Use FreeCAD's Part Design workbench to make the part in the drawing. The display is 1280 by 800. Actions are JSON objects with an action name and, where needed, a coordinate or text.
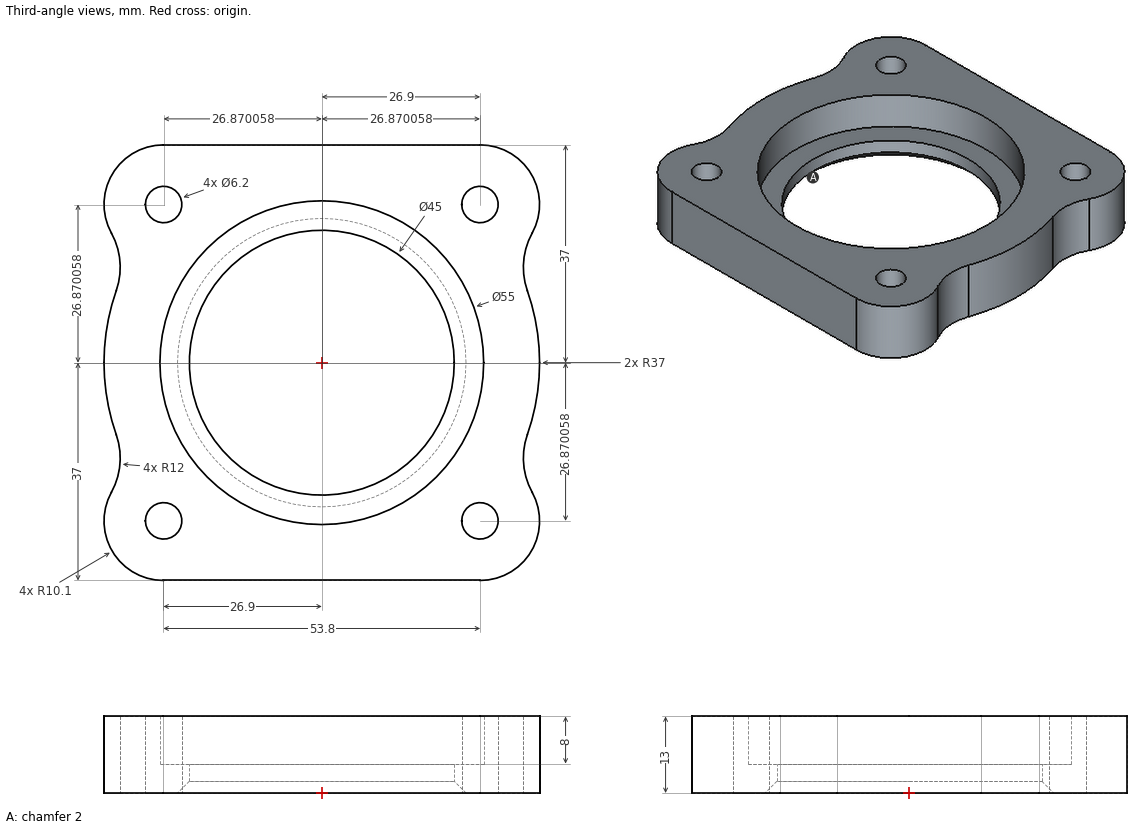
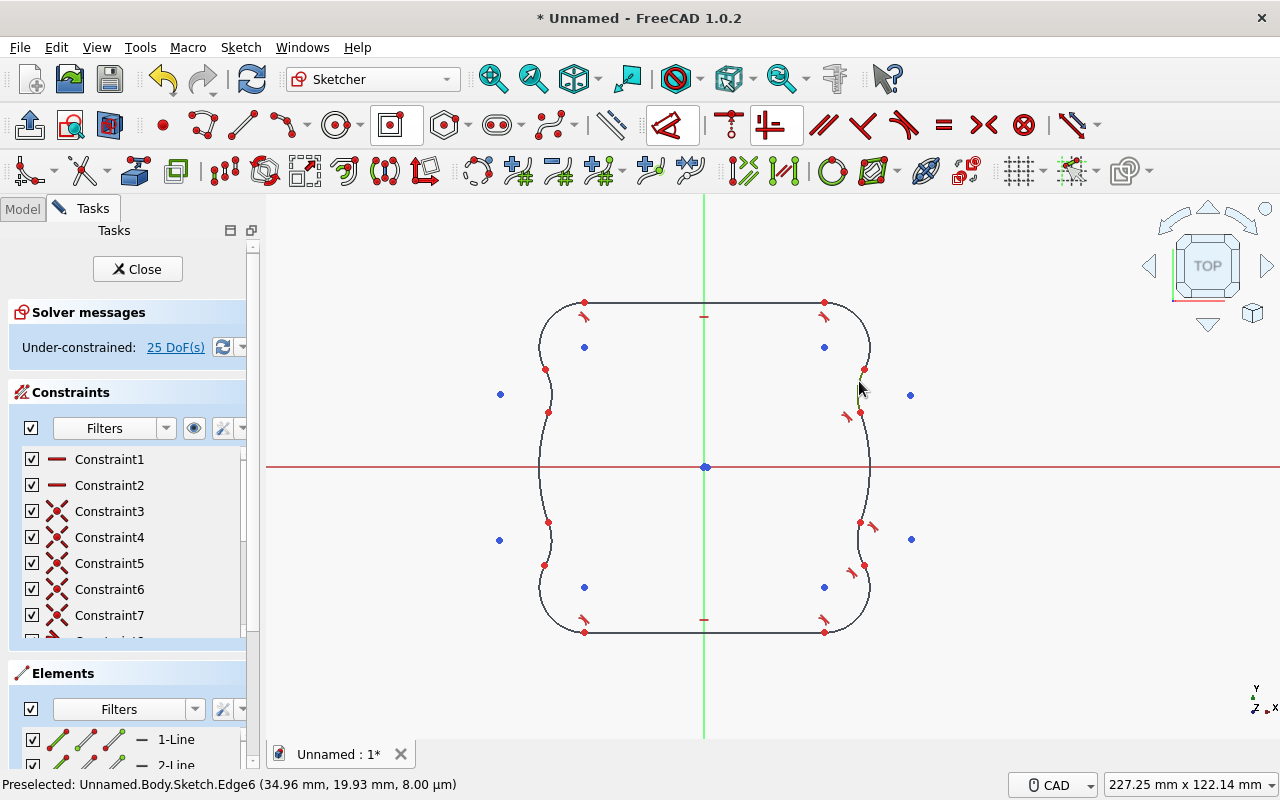
{"action": "left_click", "coordinate": [869, 342]}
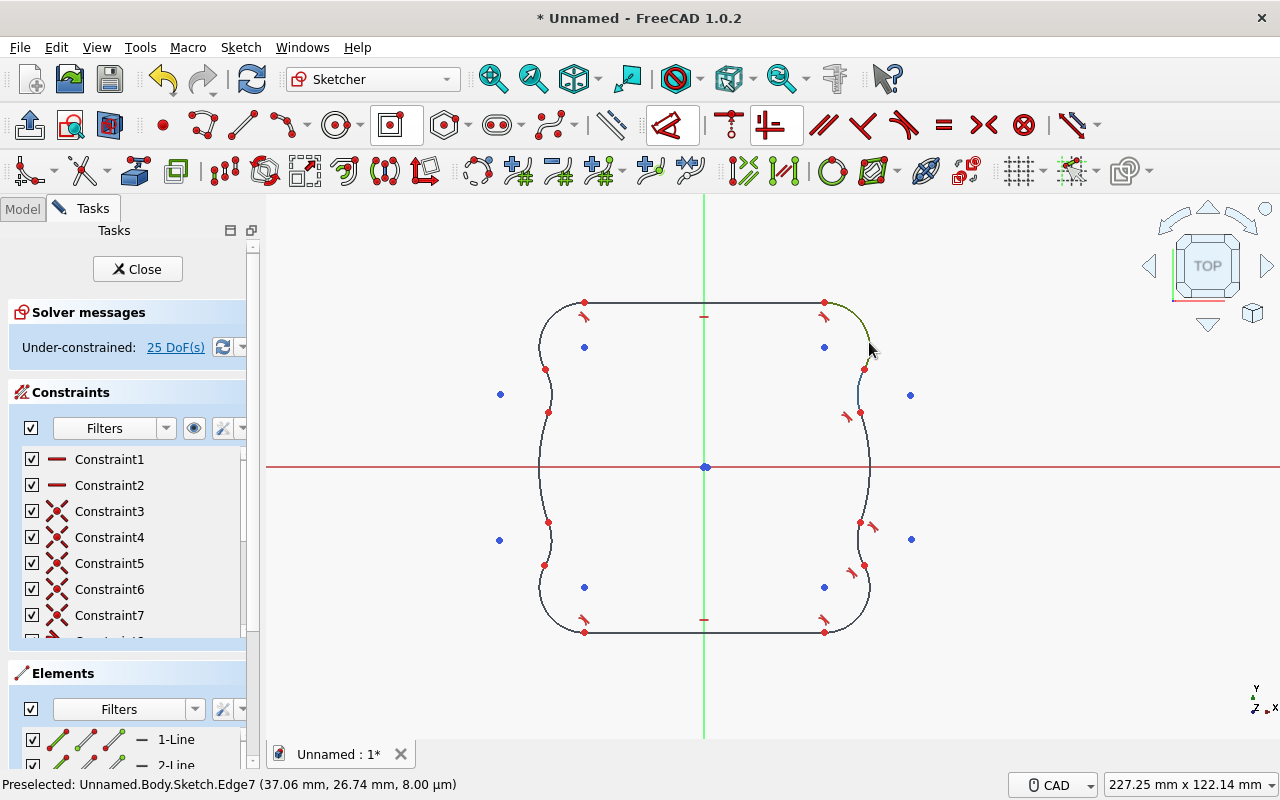
{"action": "key", "text": "t"}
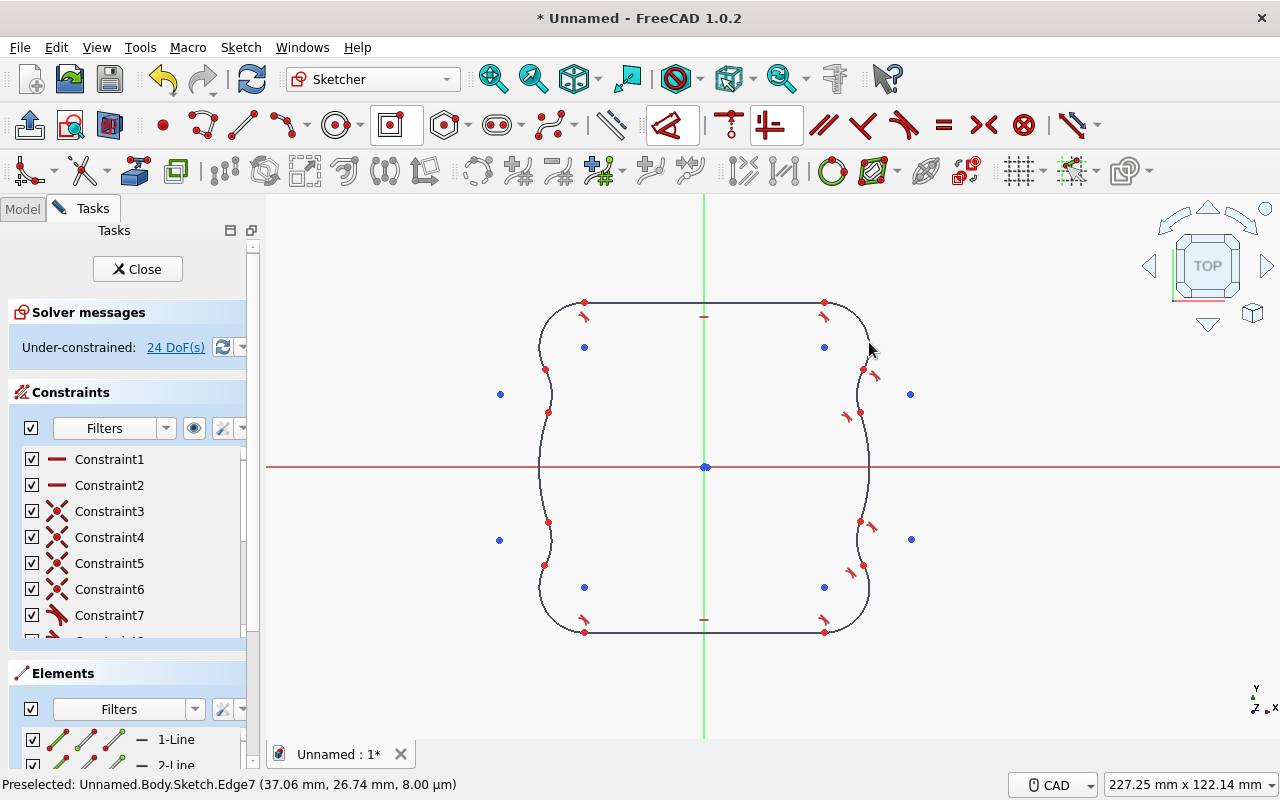
{"action": "left_click", "coordinate": [558, 311]}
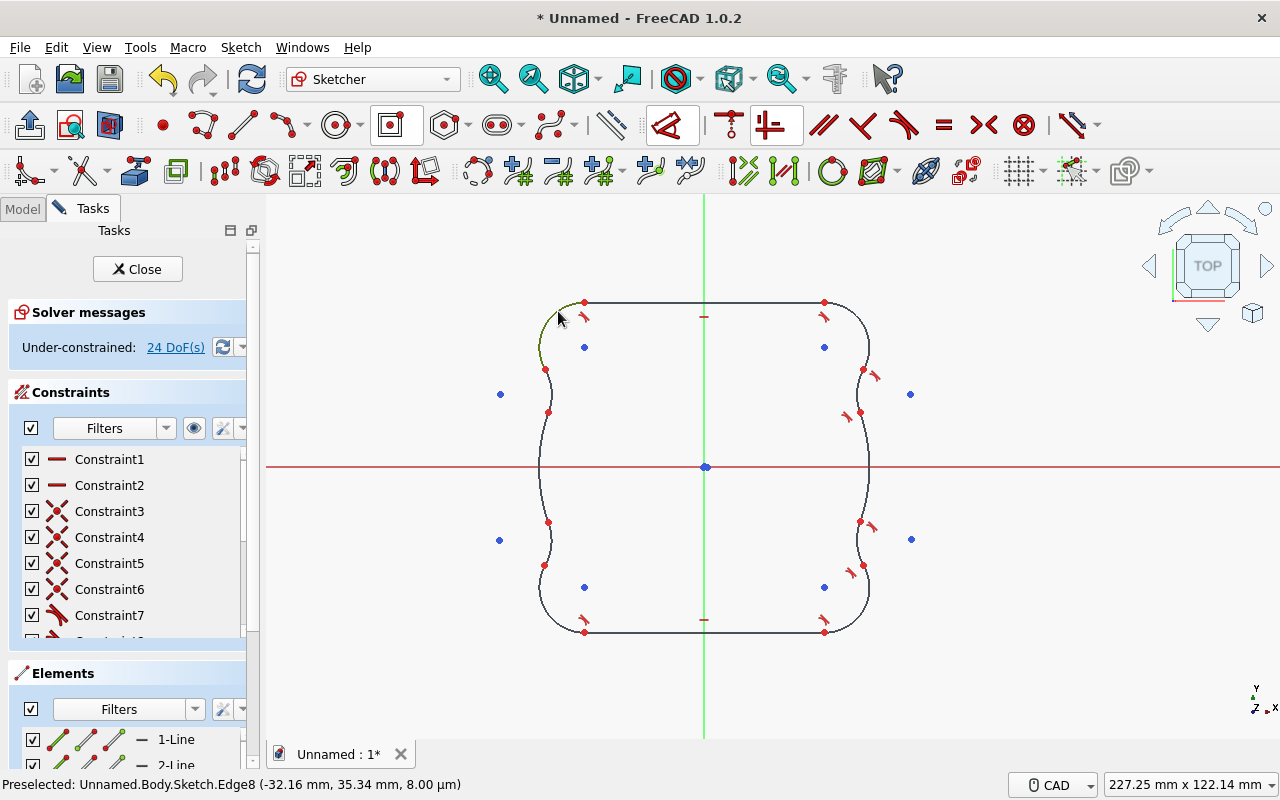
{"action": "left_click", "coordinate": [551, 400]}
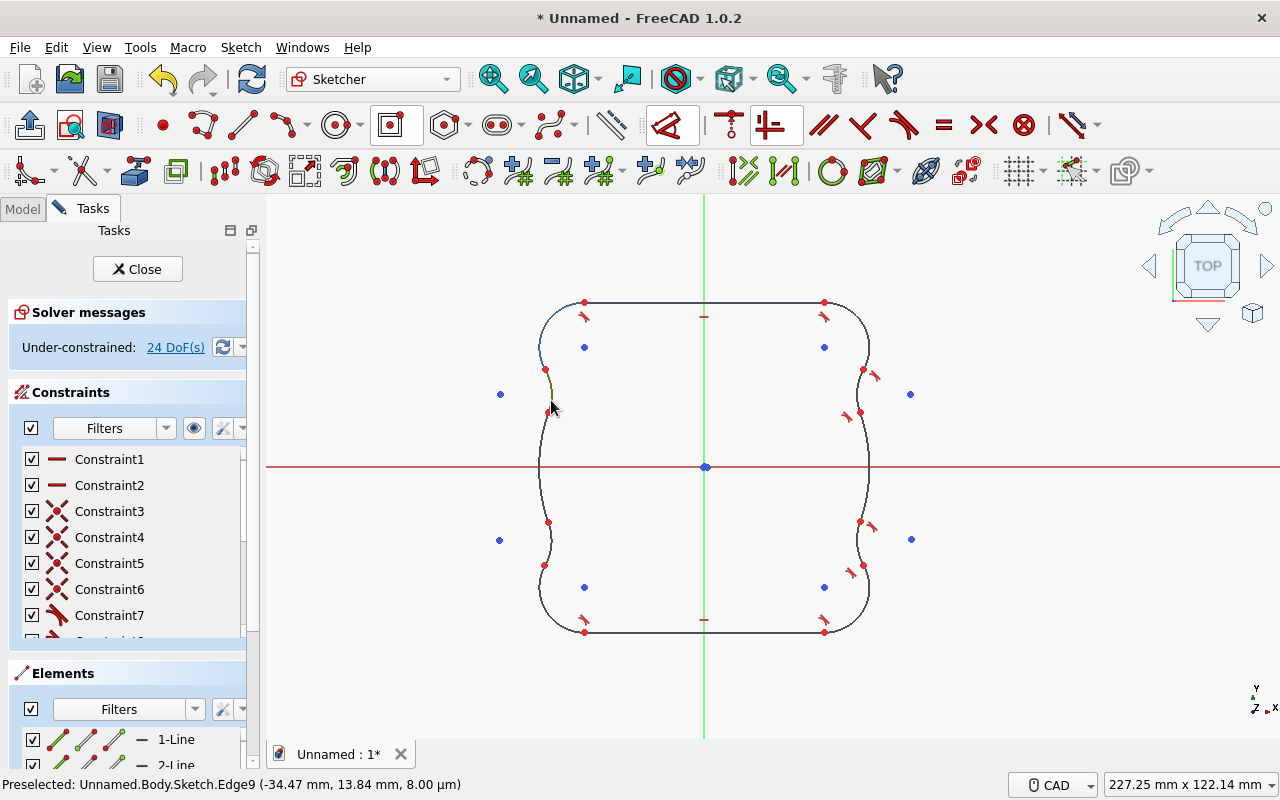
{"action": "key", "text": "t"}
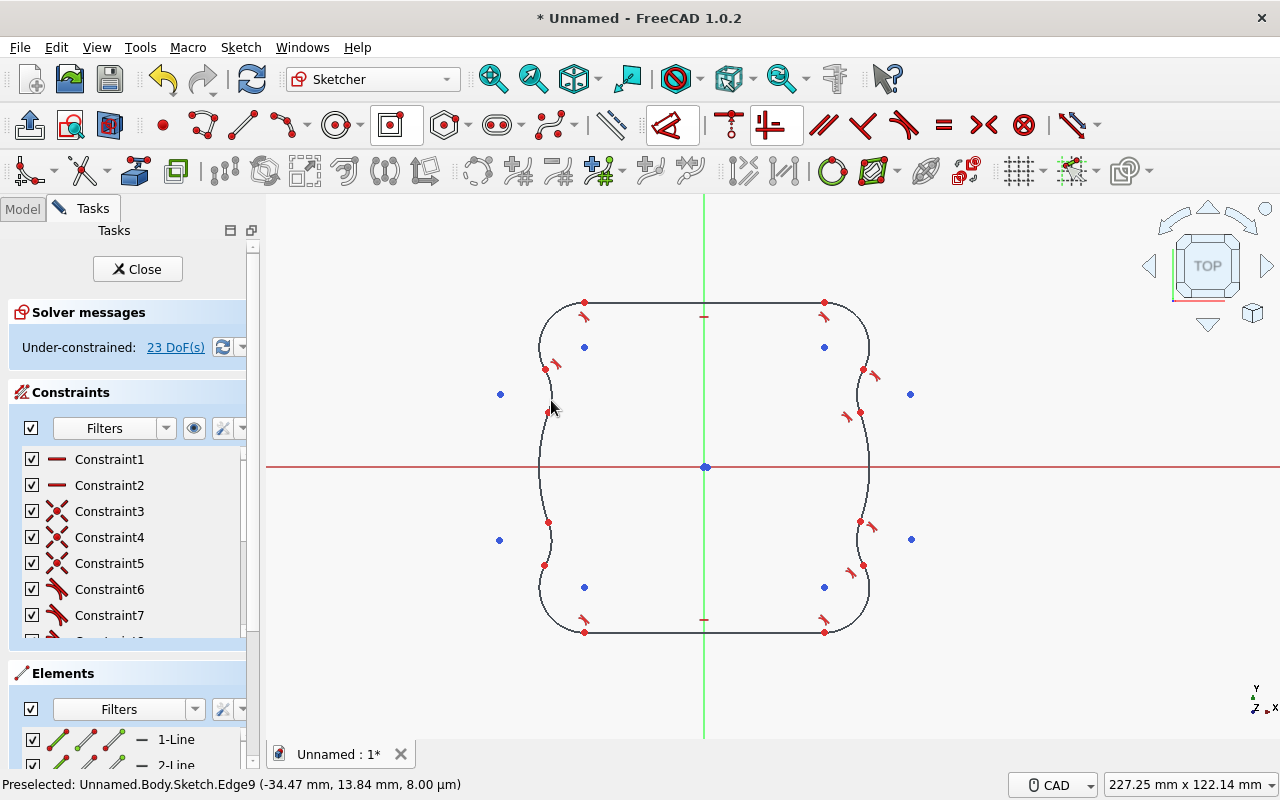
{"action": "left_click", "coordinate": [551, 400]}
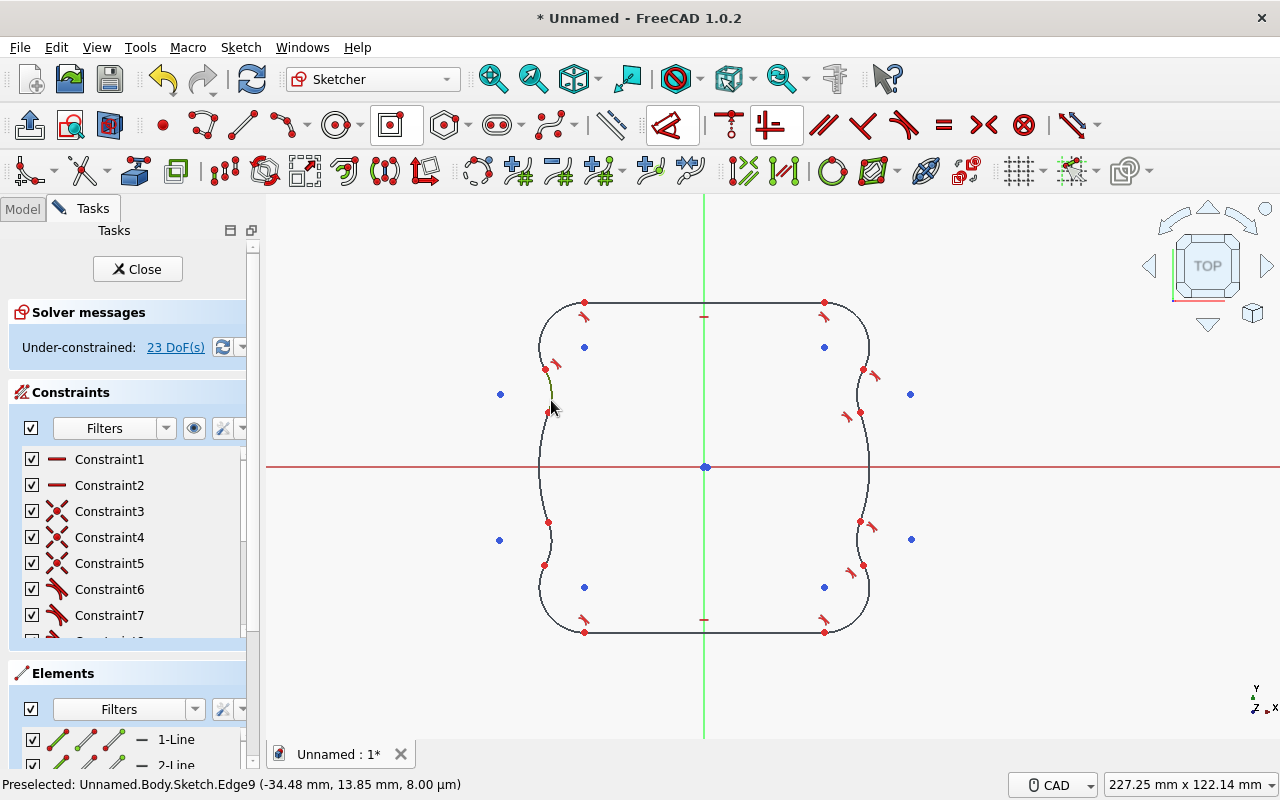
{"action": "left_click", "coordinate": [541, 446]}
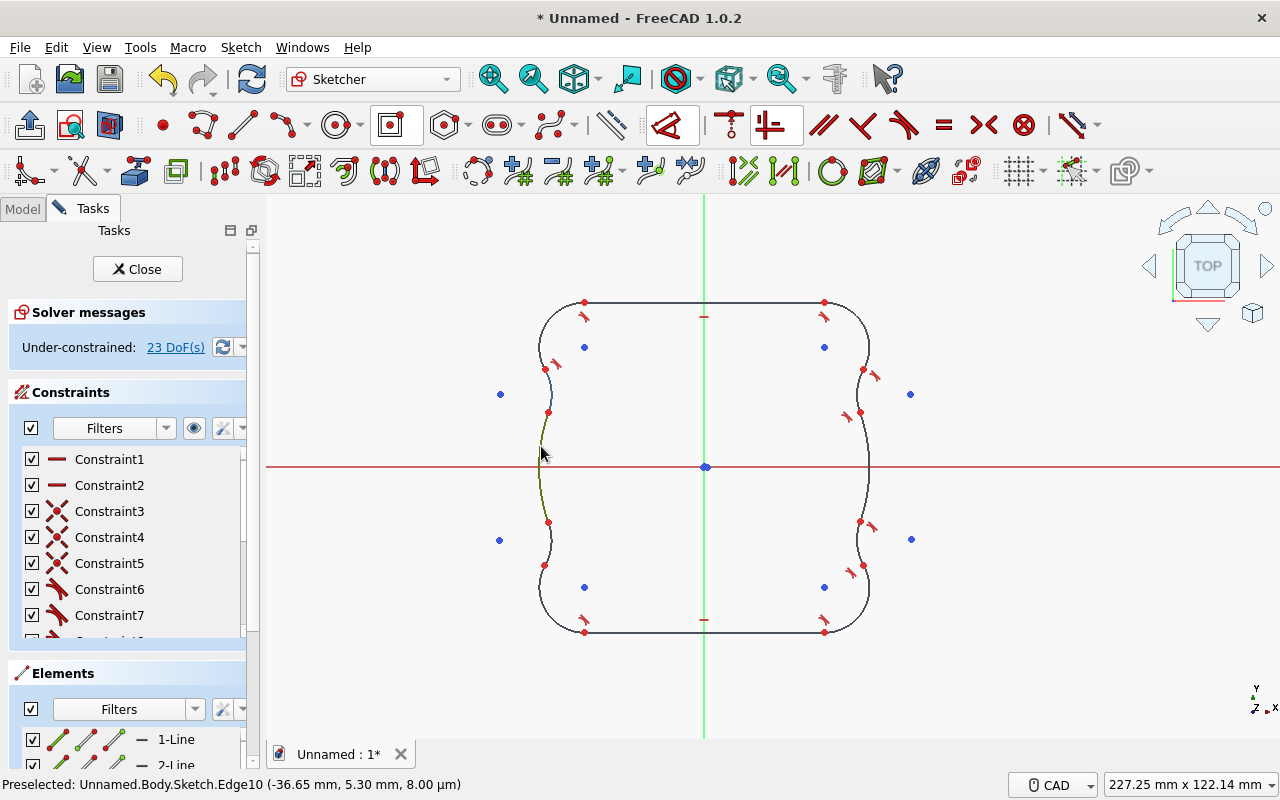
{"action": "key", "text": "t"}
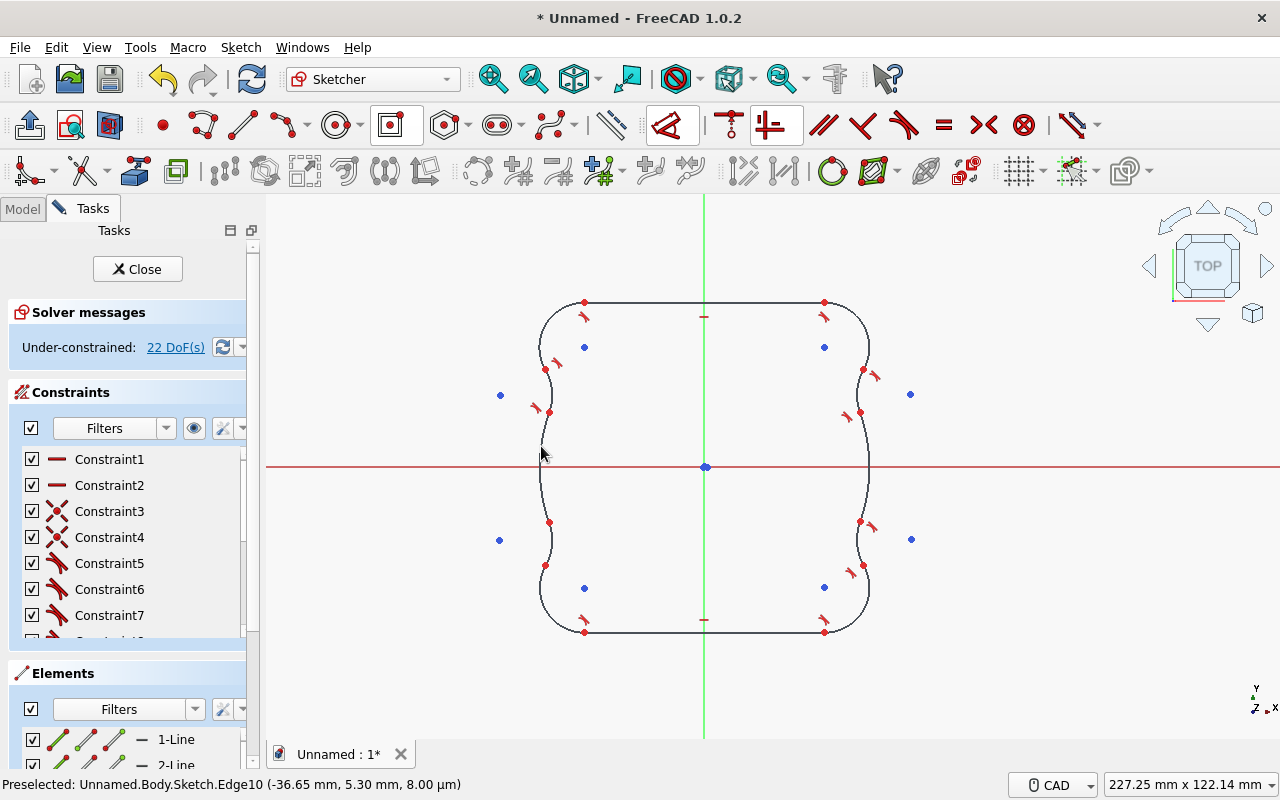
{"action": "left_click", "coordinate": [541, 445]}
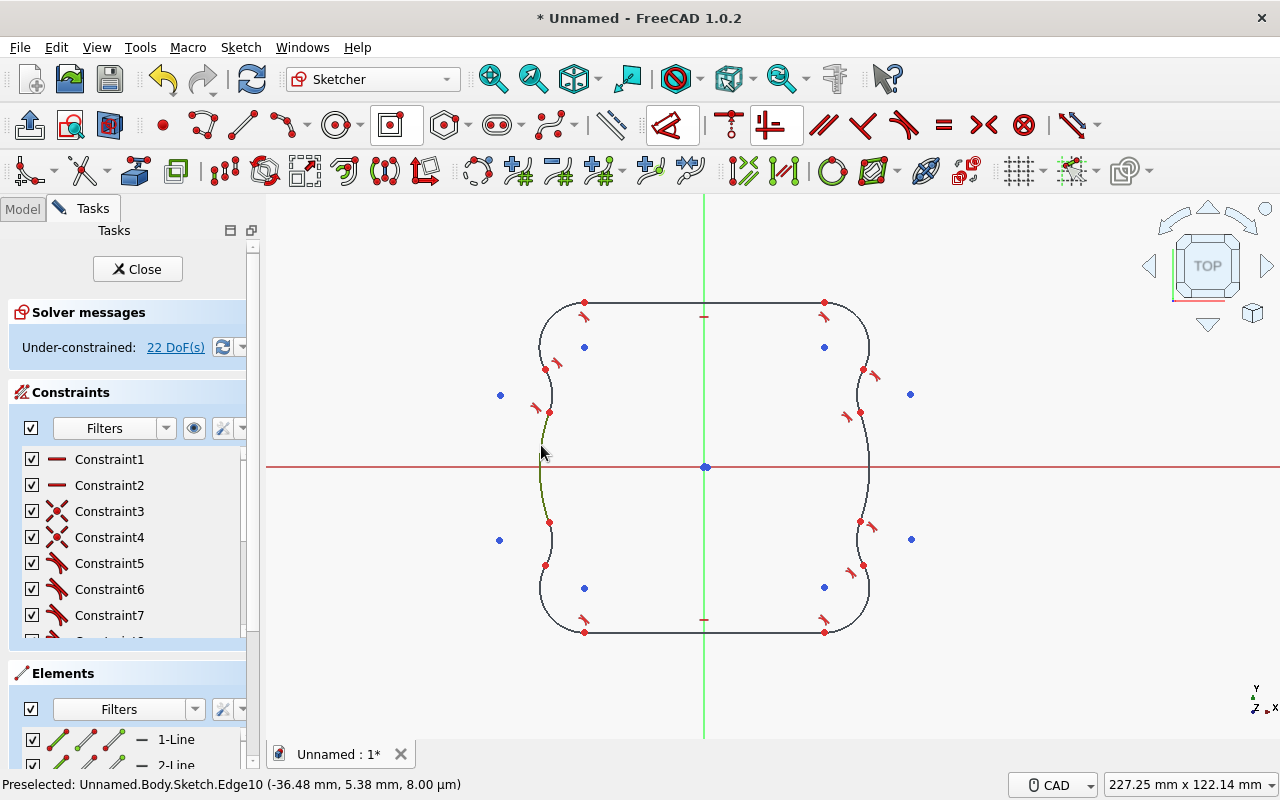
{"action": "left_click", "coordinate": [551, 553]}